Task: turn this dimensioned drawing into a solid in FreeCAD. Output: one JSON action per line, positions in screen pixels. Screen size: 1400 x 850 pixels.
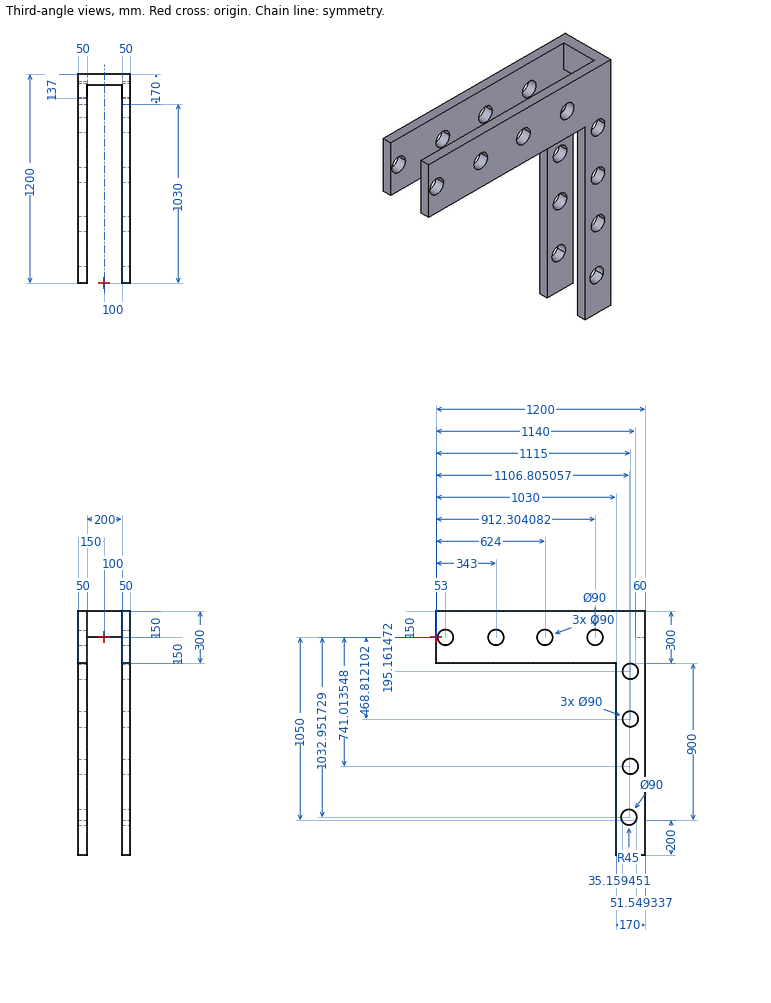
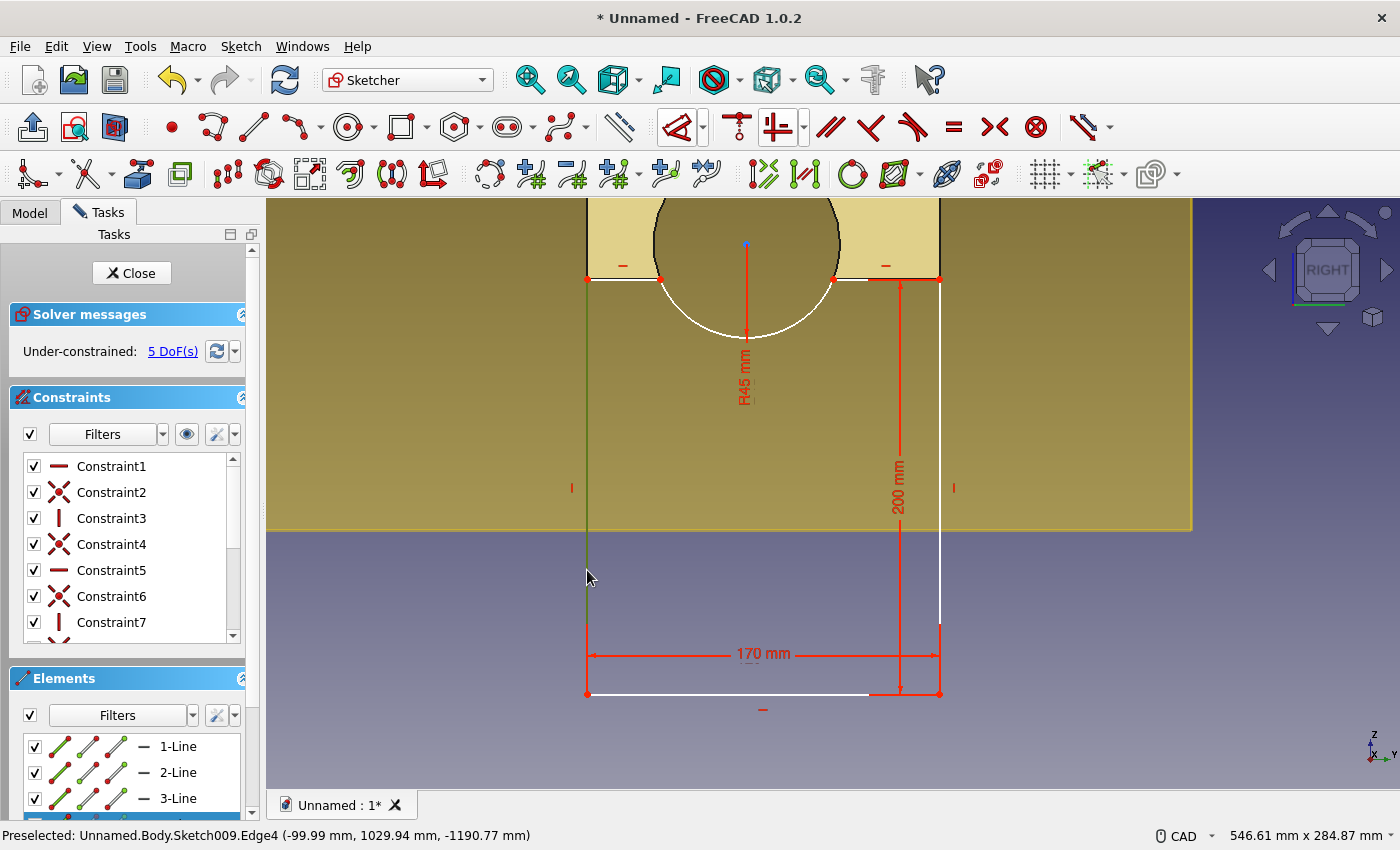
{"action": "left_click", "coordinate": [702, 128]}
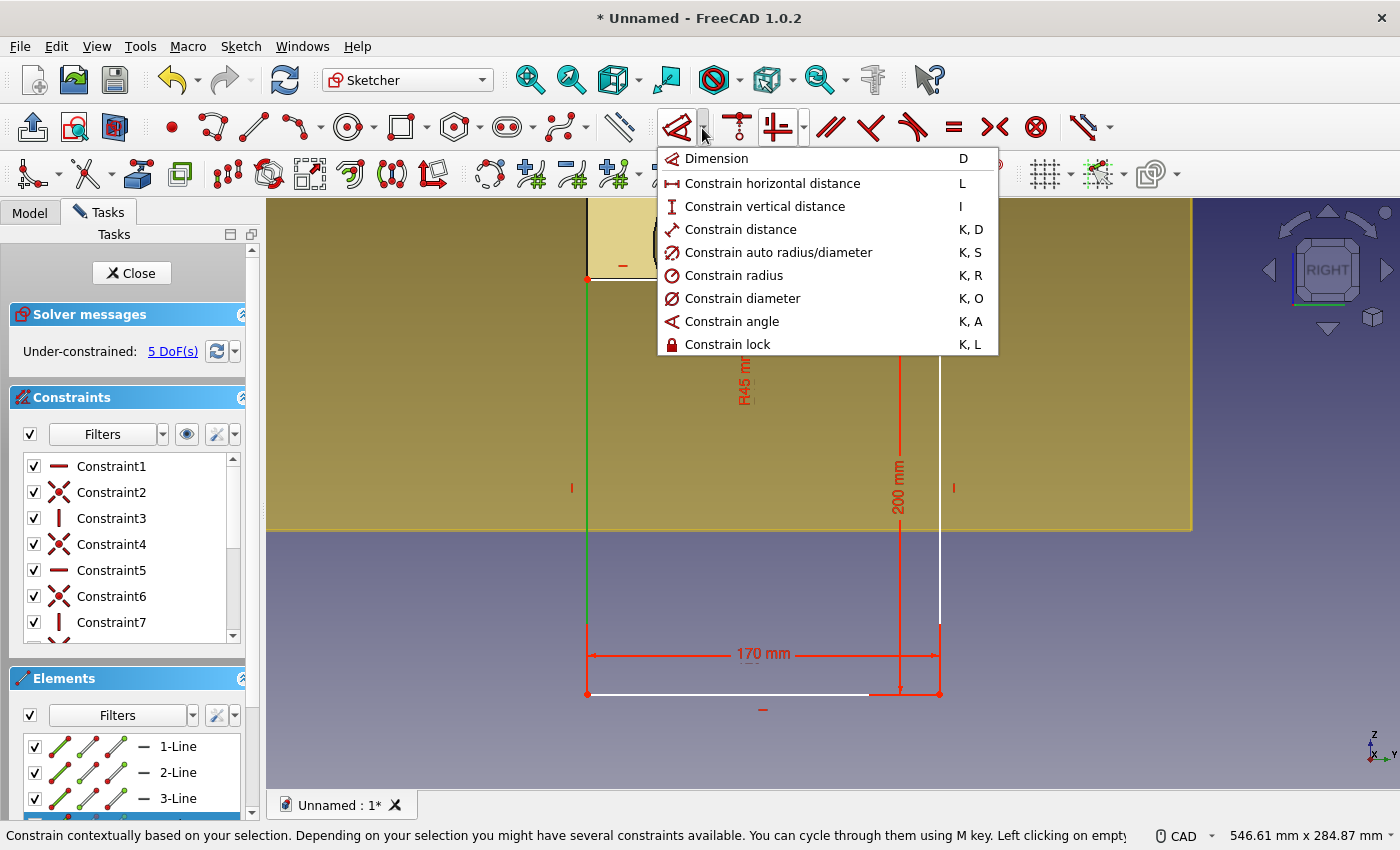
{"action": "left_click", "coordinate": [828, 206]}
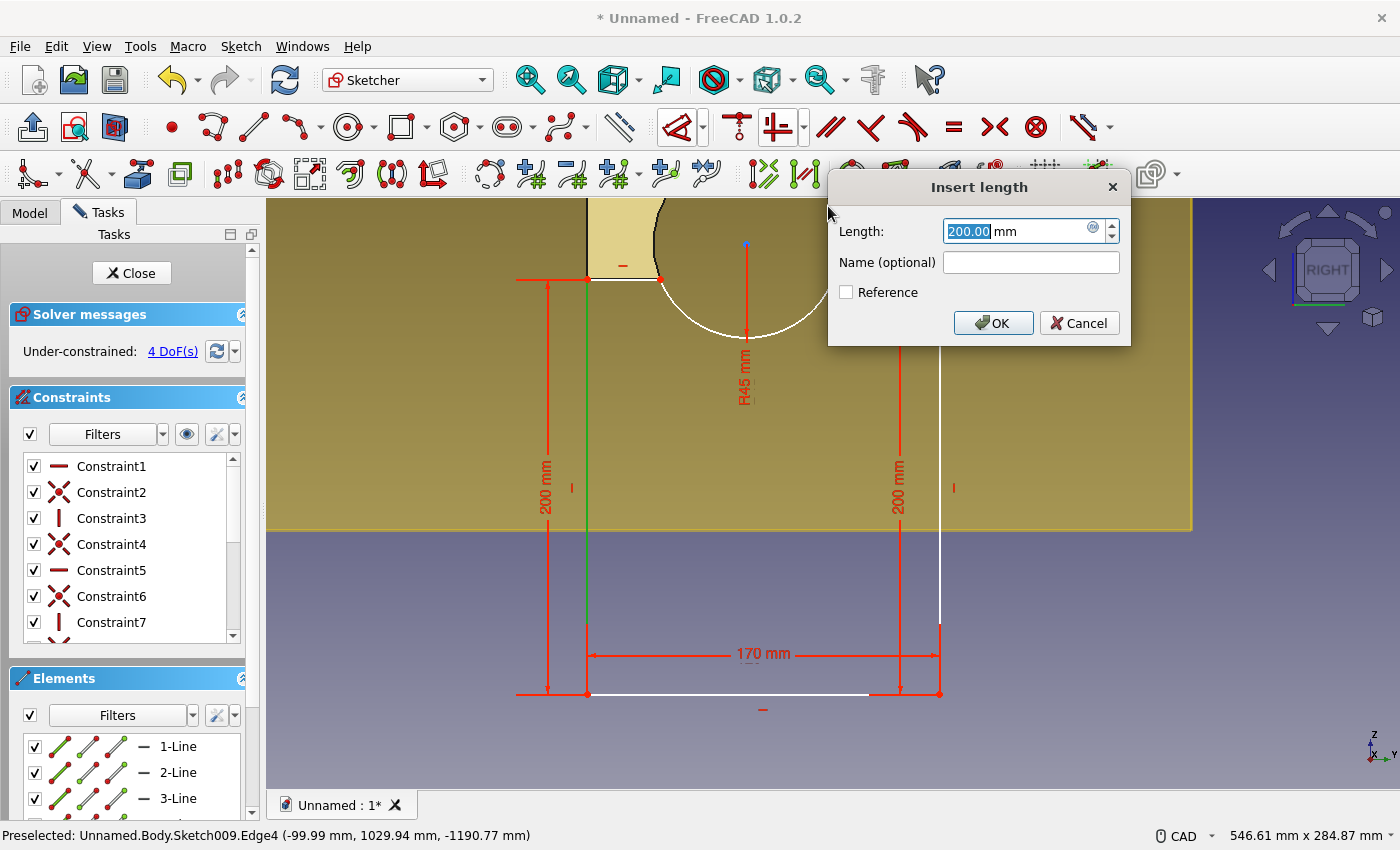
{"action": "type", "text": "200"}
{"action": "key", "text": "Return"}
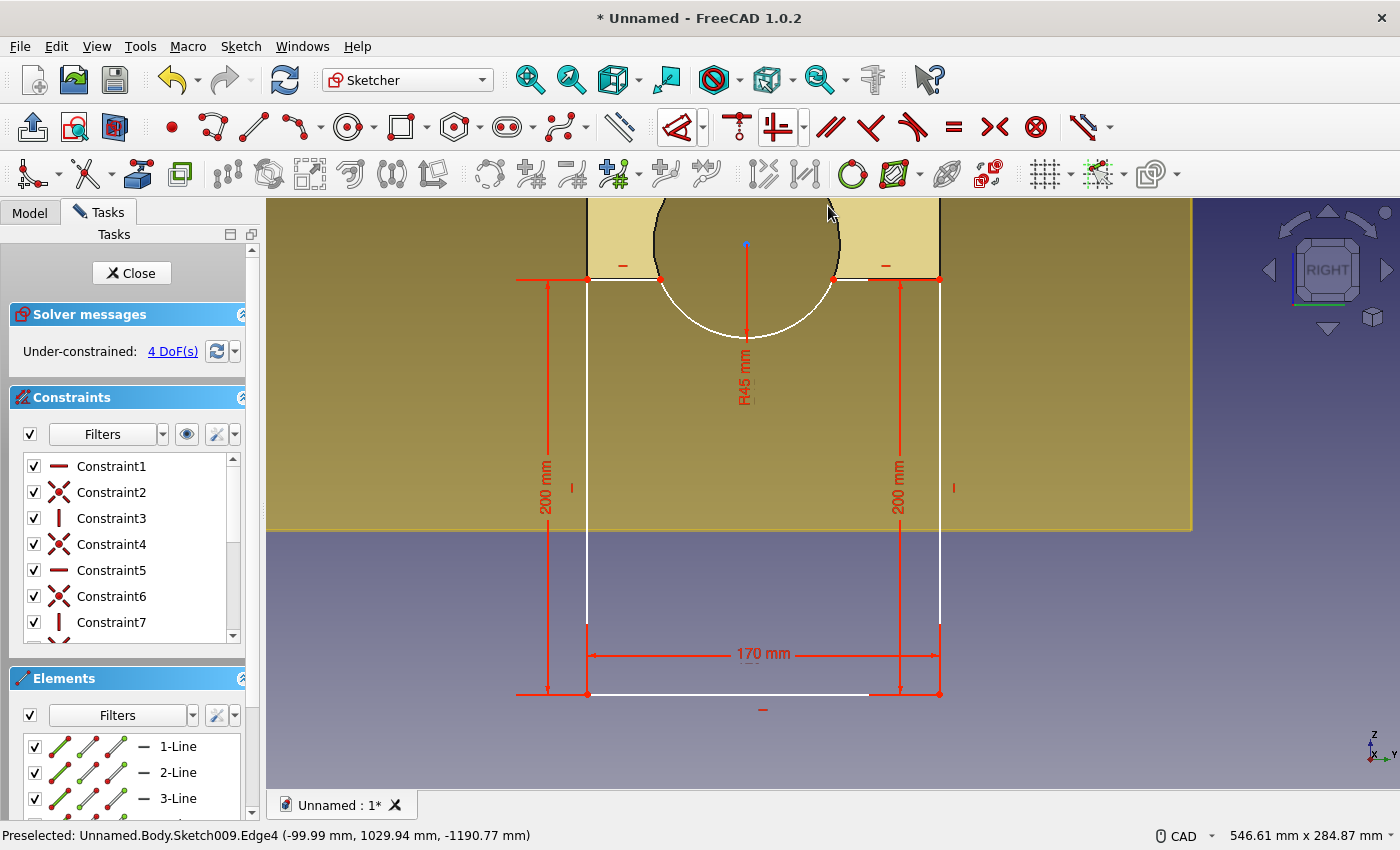
{"action": "left_click", "coordinate": [833, 280]}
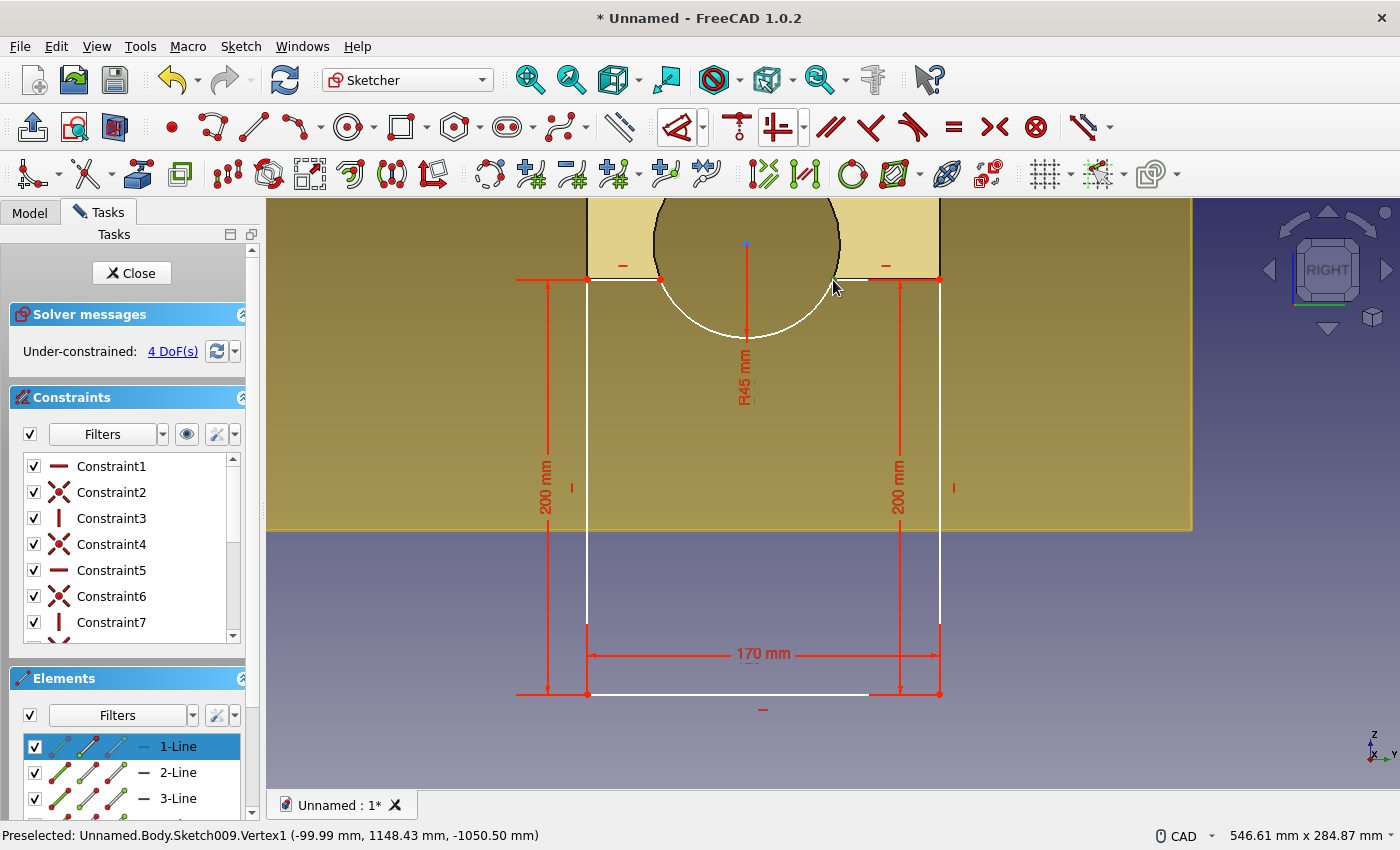
{"action": "key", "text": "i"}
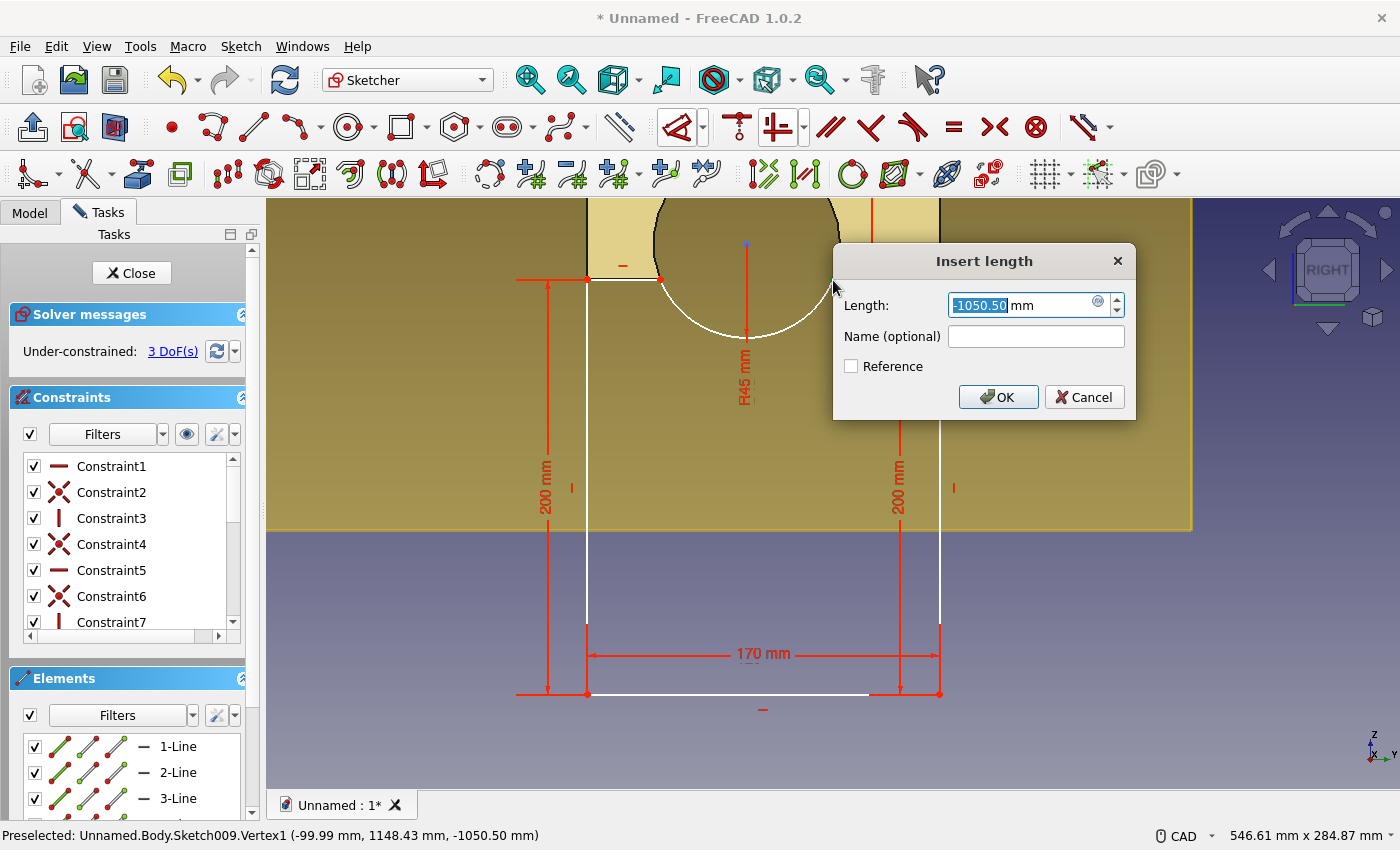
{"action": "type", "text": "-1050"}
{"action": "key", "text": "Return"}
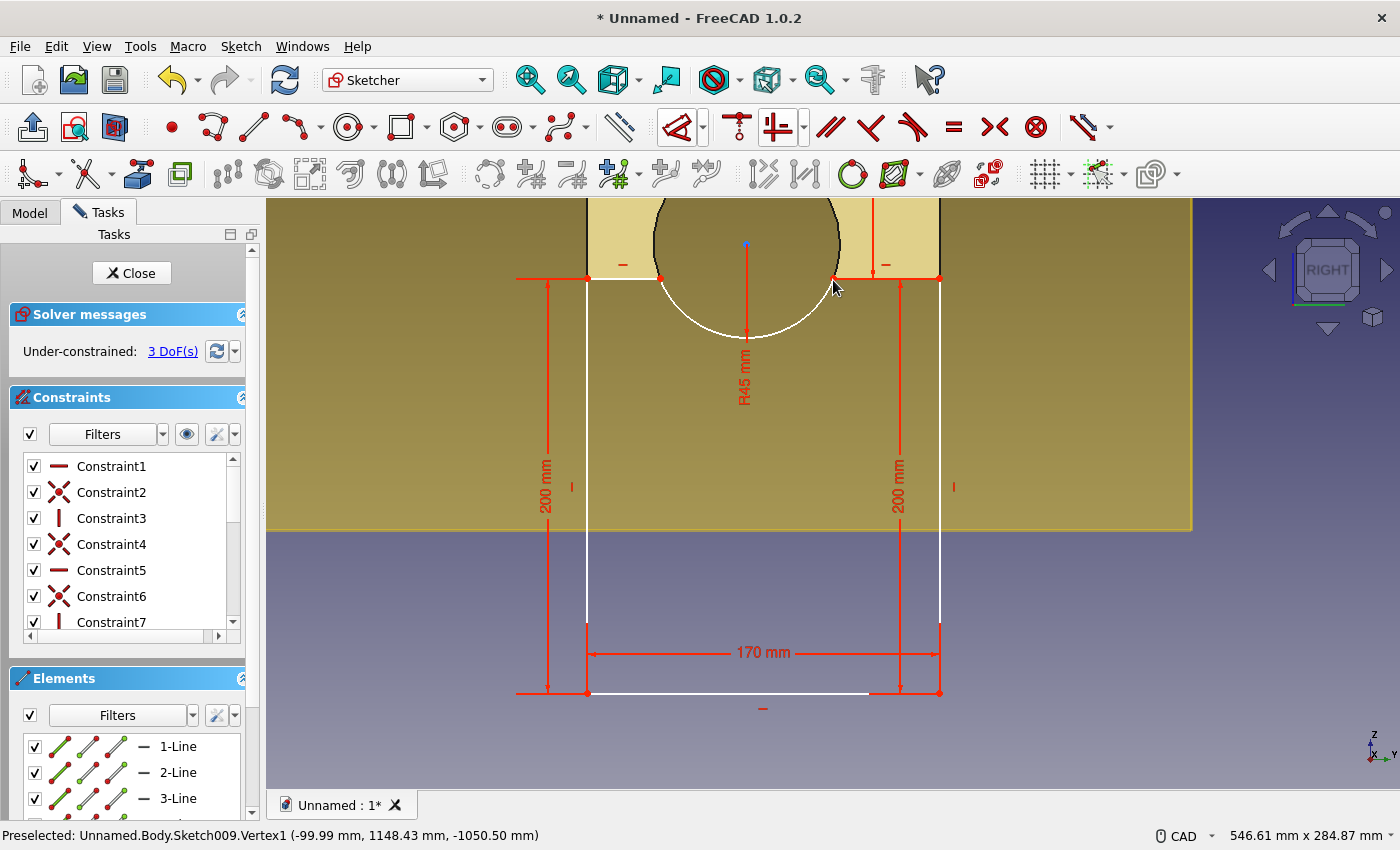
{"action": "left_click", "coordinate": [940, 279]}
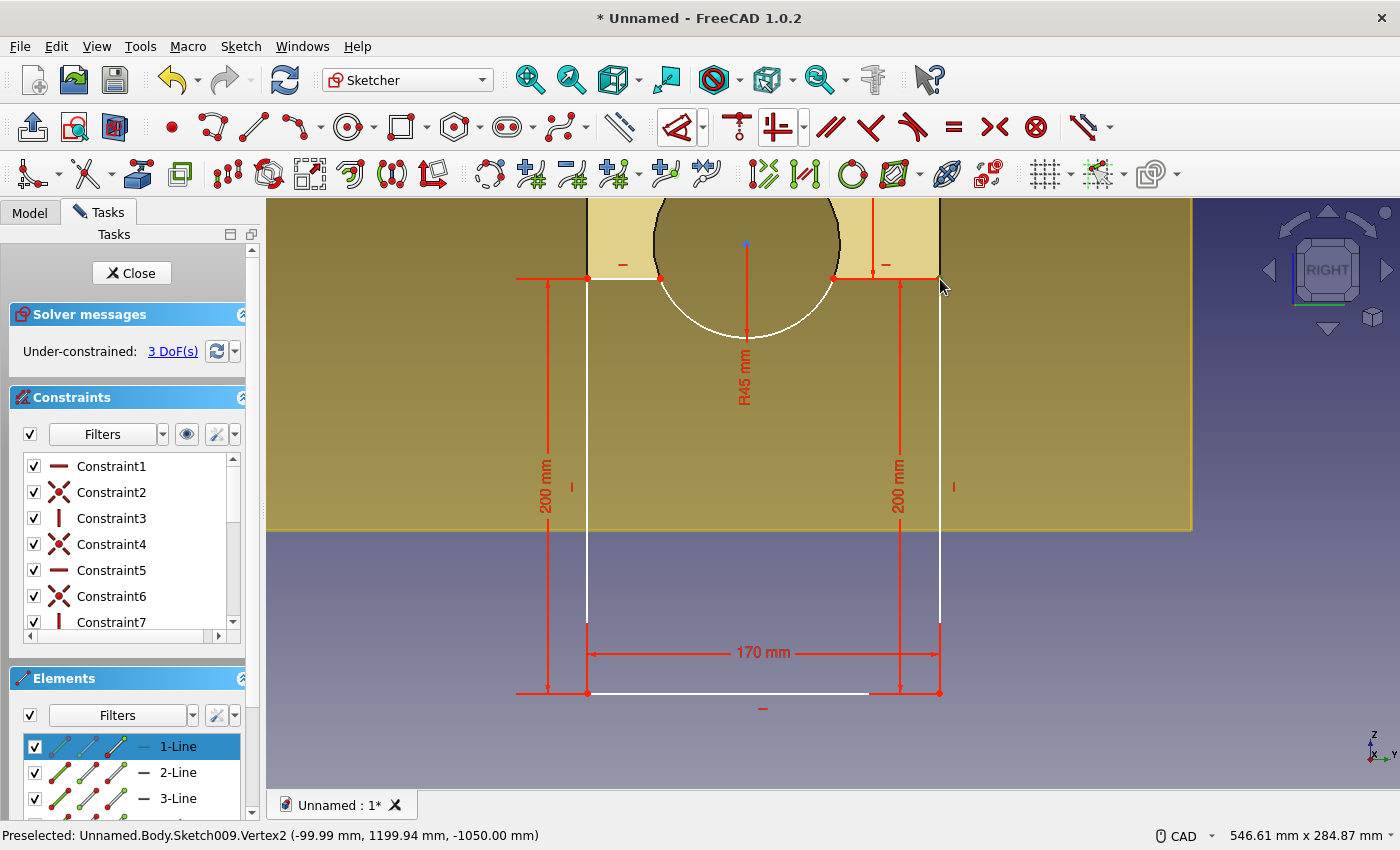
{"action": "left_click", "coordinate": [702, 128]}